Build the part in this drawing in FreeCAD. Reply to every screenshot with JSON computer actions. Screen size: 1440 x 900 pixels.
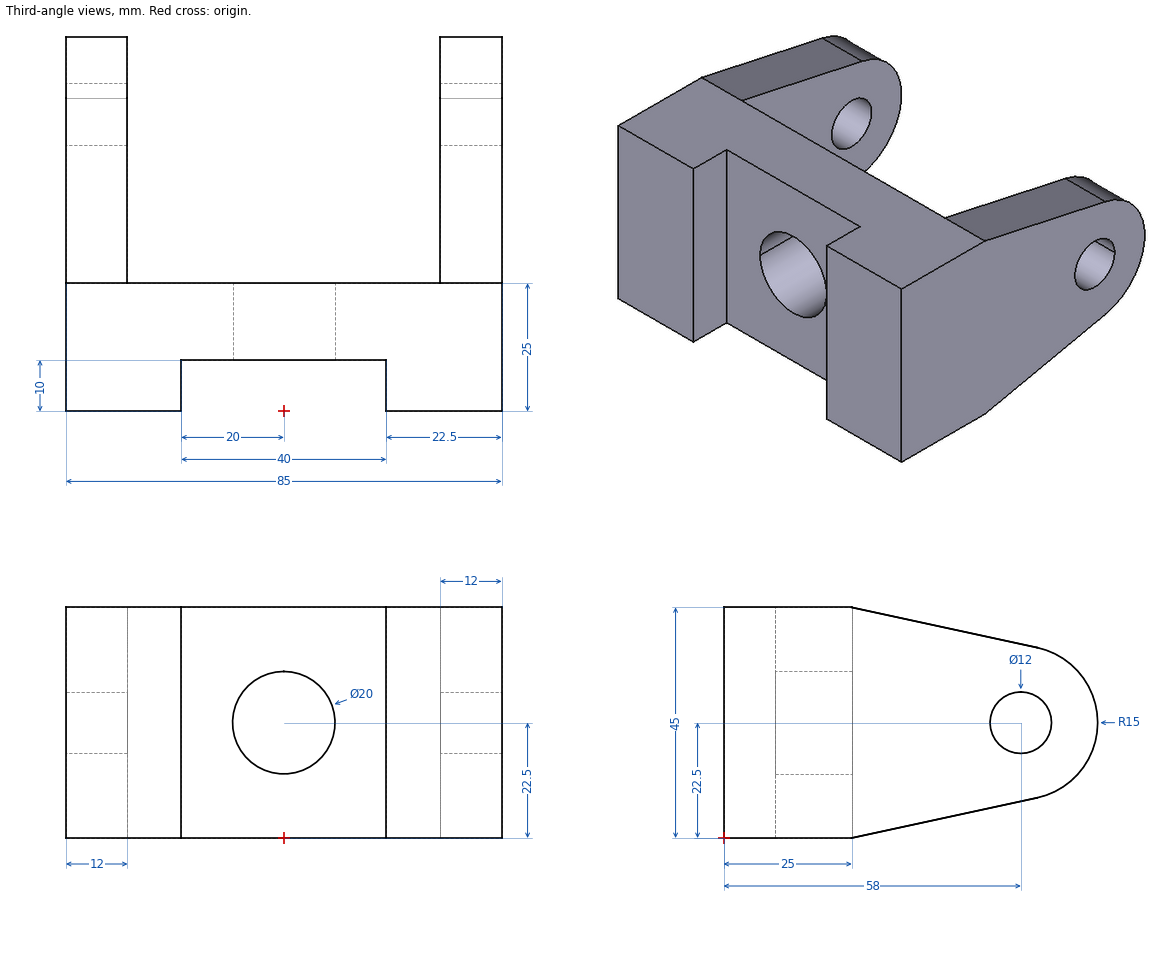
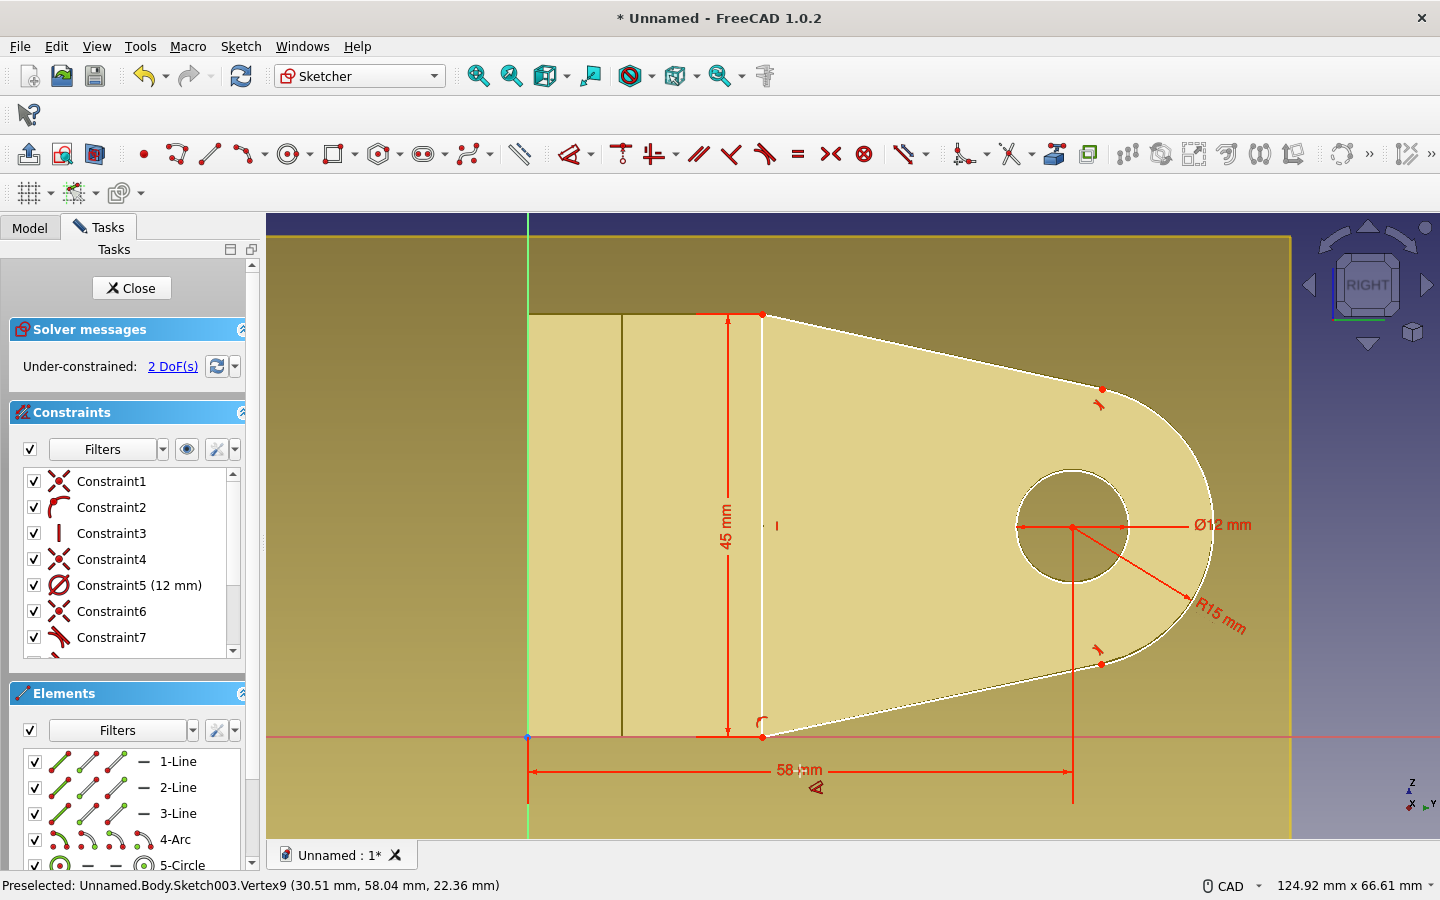
{"action": "left_click", "coordinate": [762, 314]}
{"action": "left_click", "coordinate": [645, 771]}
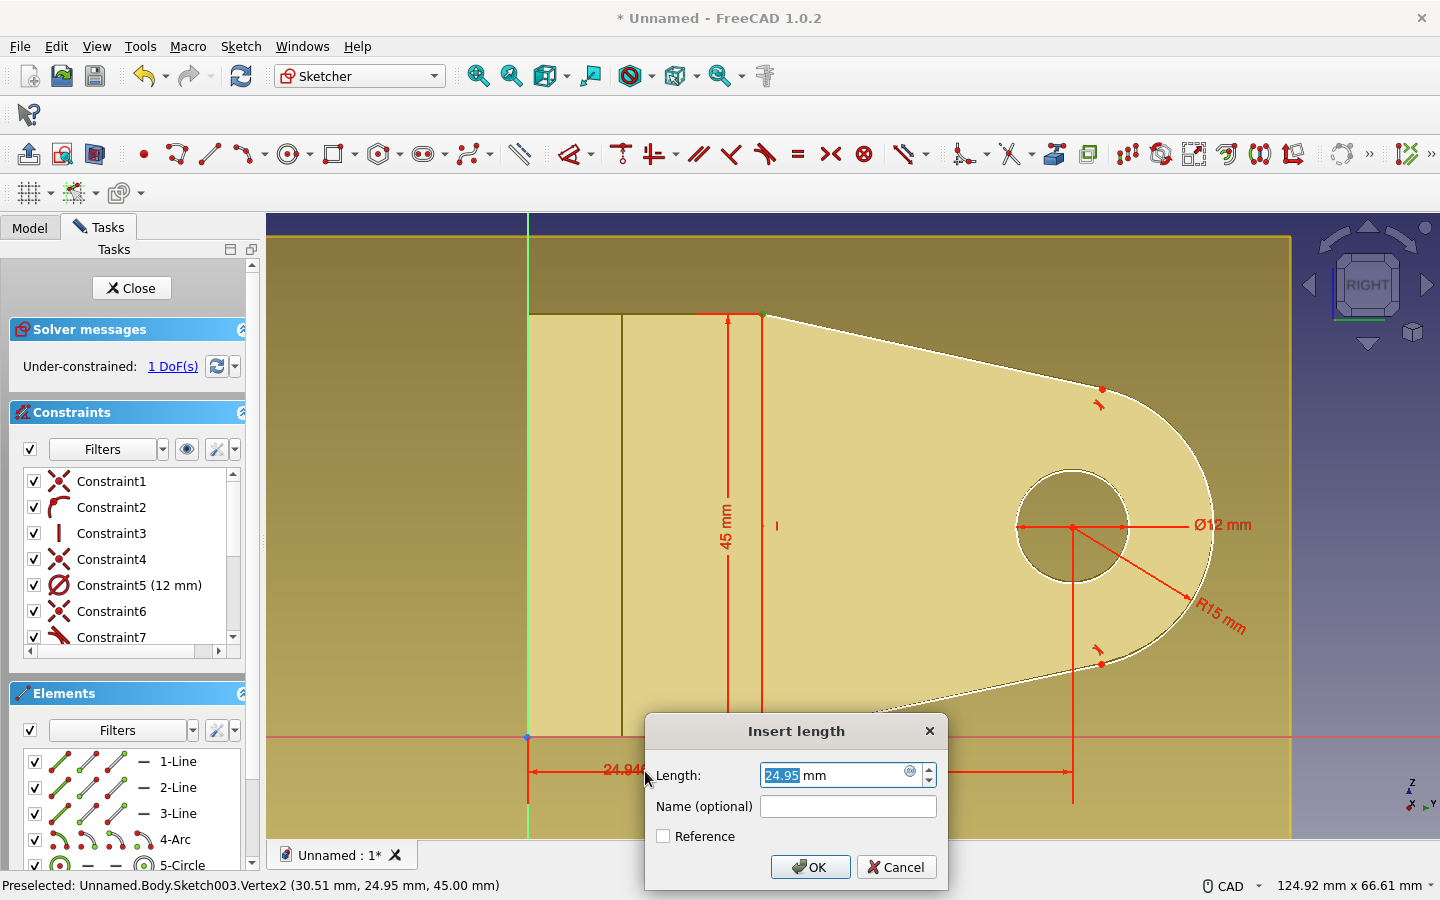
{"action": "type", "text": "25"}
{"action": "key", "text": "Return"}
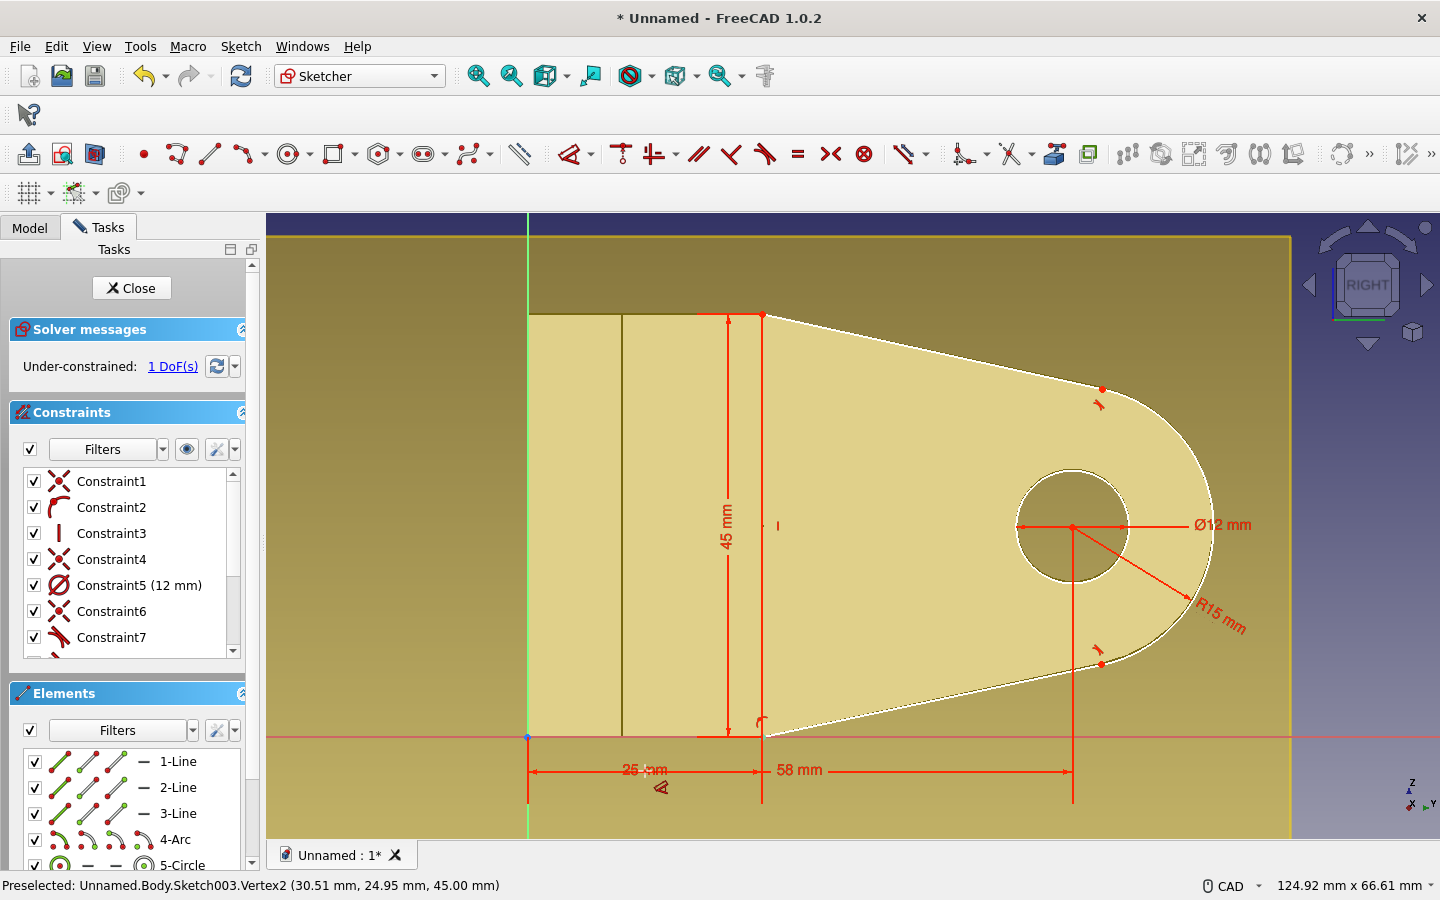
{"action": "left_click", "coordinate": [1073, 527]}
{"action": "left_click", "coordinate": [494, 632]}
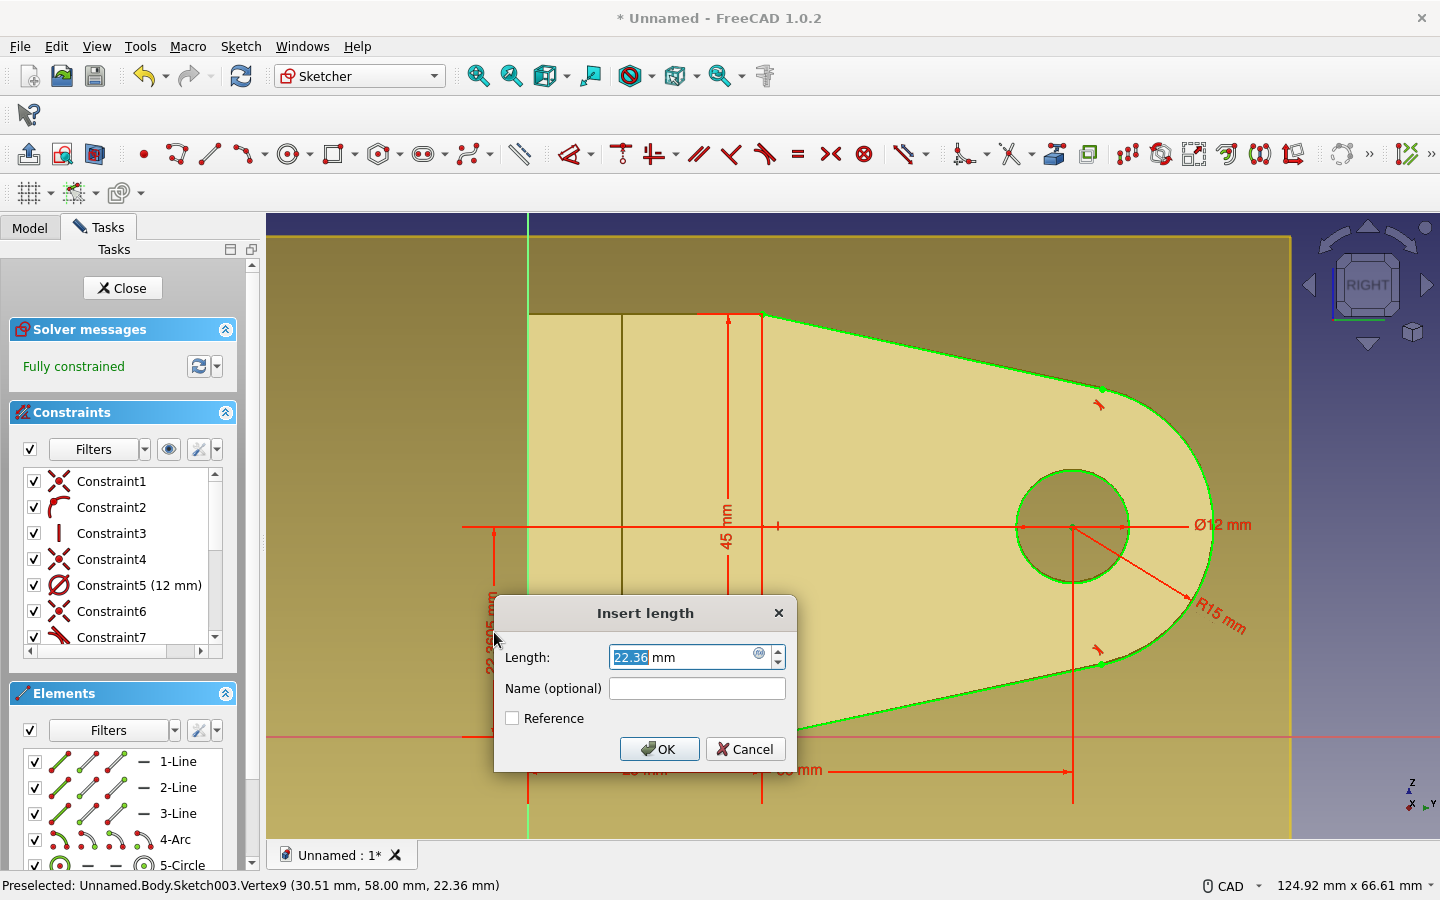
{"action": "type", "text": "22.5"}
{"action": "key", "text": "Return"}
{"action": "key", "text": "Escape"}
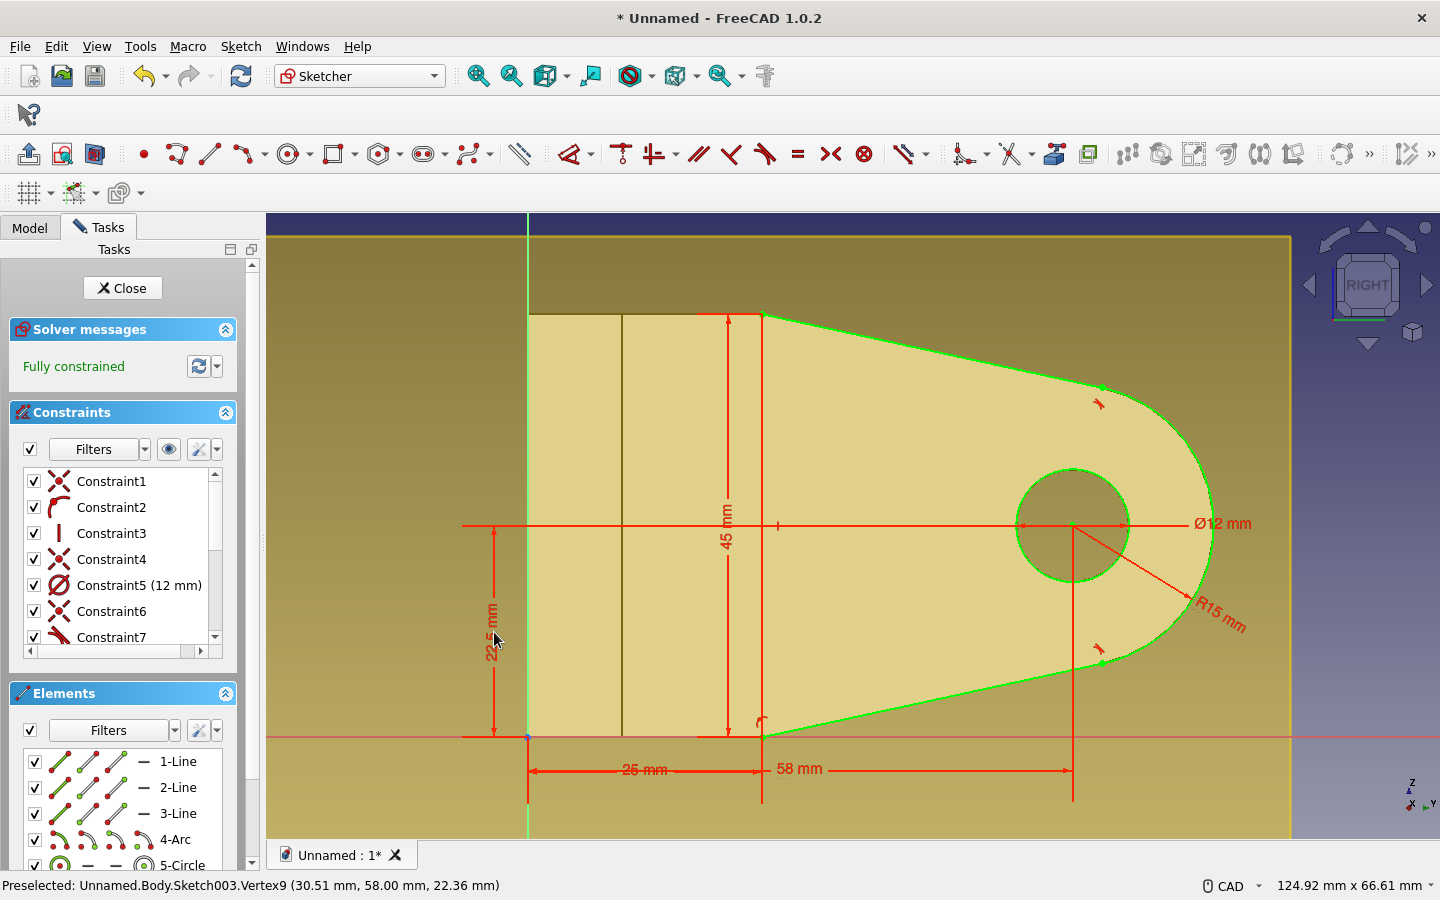
{"action": "left_click", "coordinate": [123, 288]}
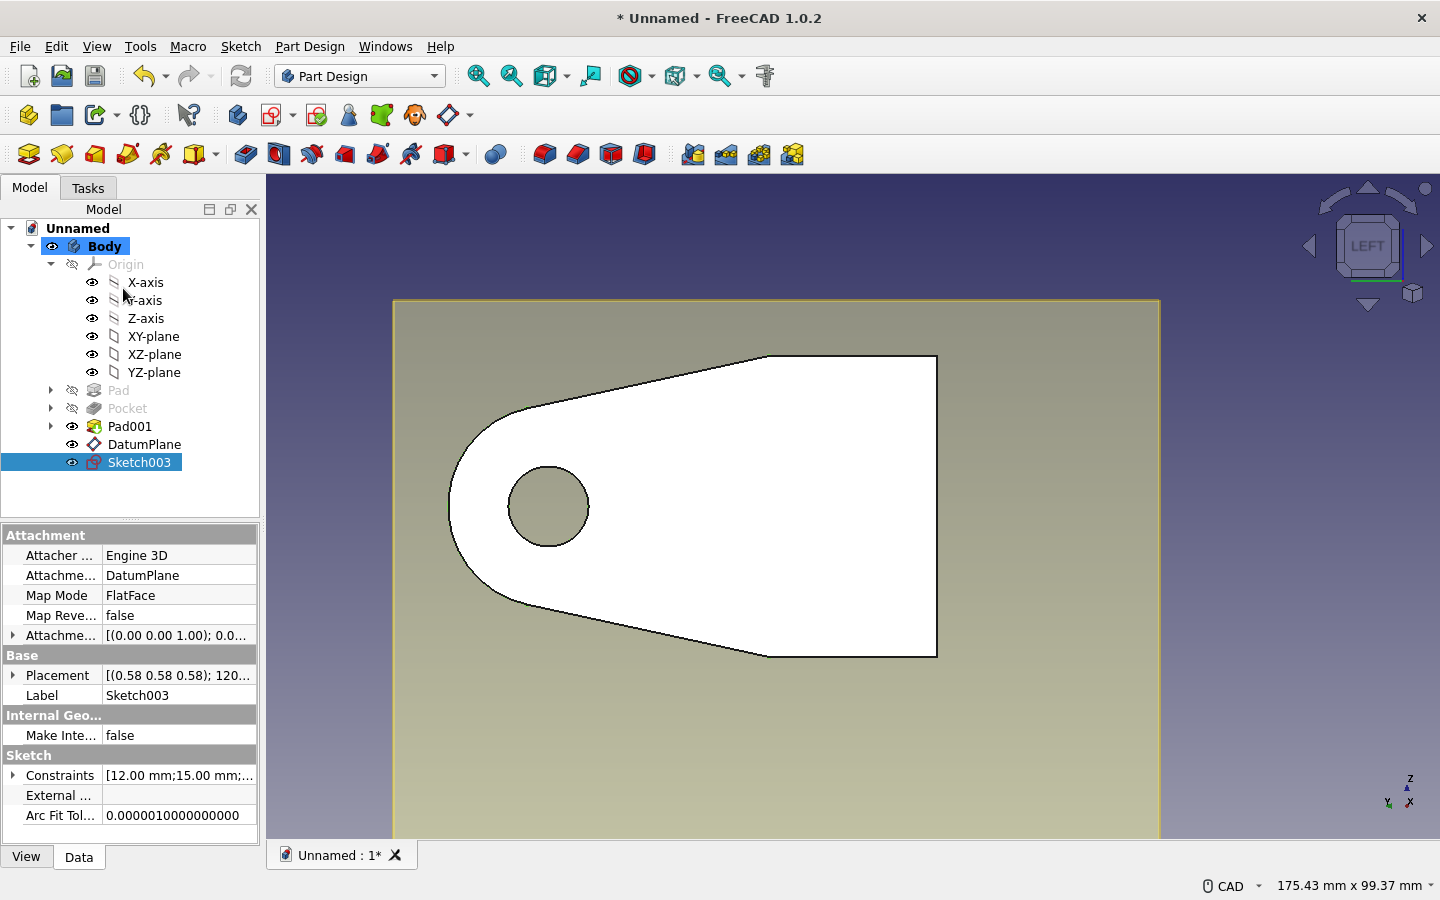
{"action": "left_click", "coordinate": [29, 154]}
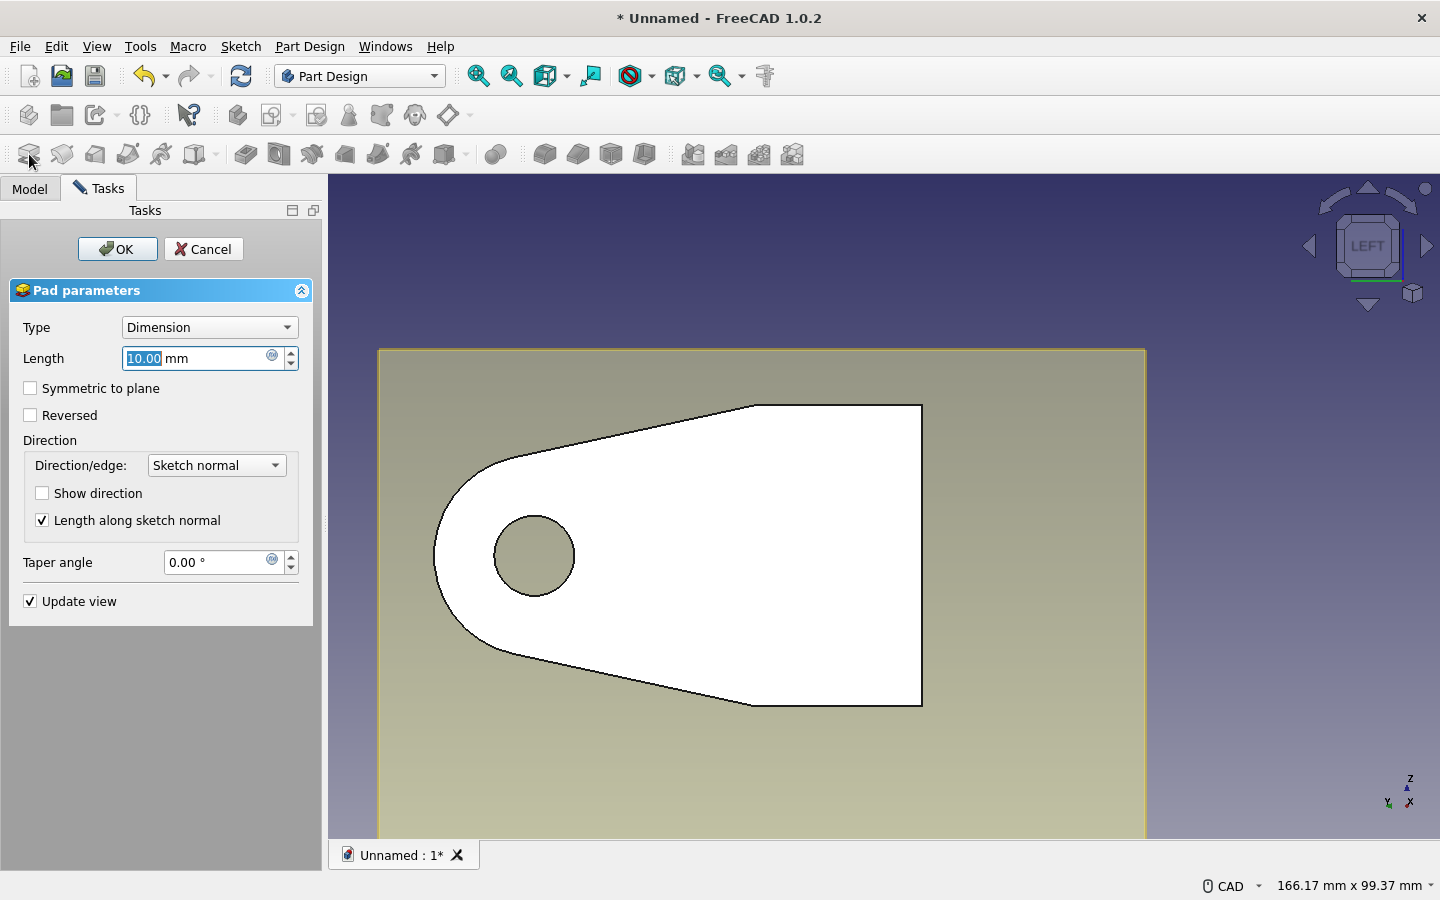
{"action": "type", "text": "12"}
{"action": "key", "text": "Tab"}